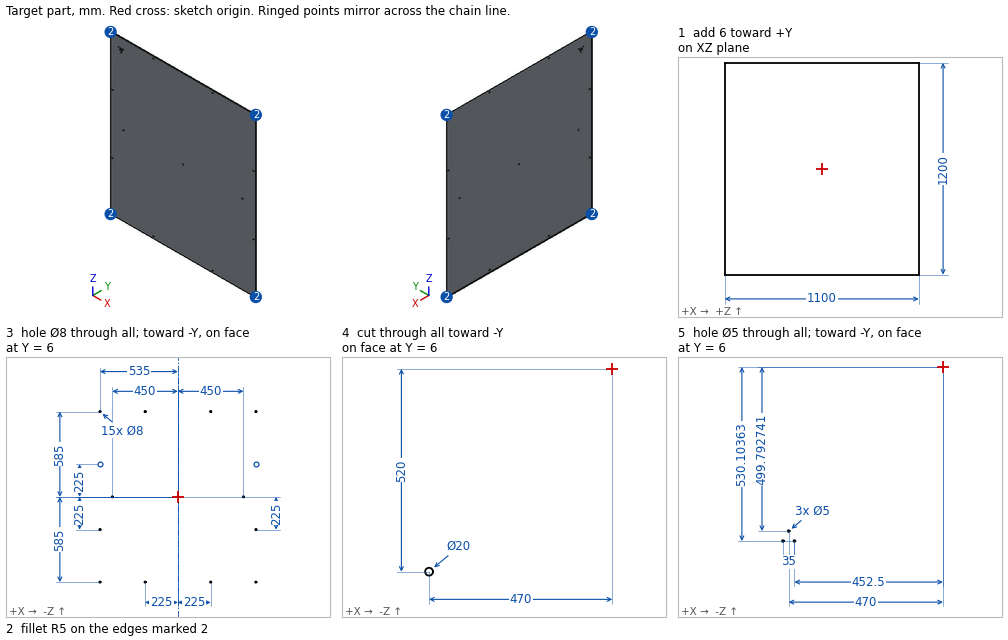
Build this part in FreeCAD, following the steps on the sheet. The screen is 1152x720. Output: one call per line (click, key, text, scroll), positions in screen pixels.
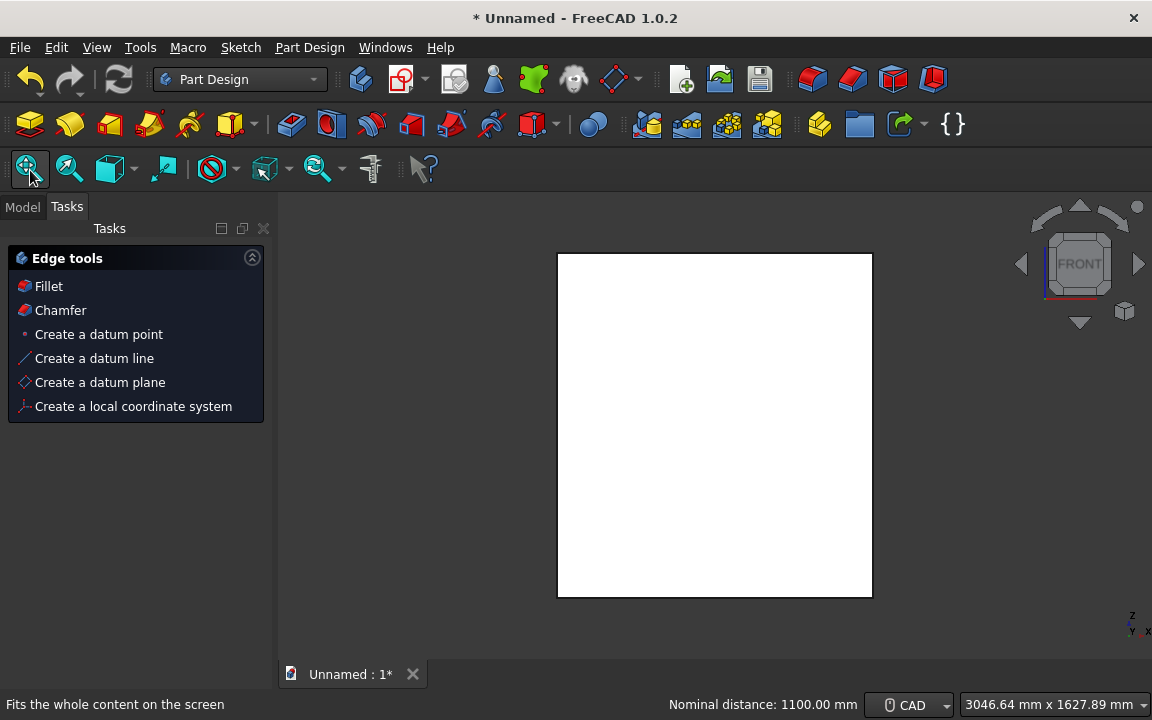
scroll(557, 597, up, 15)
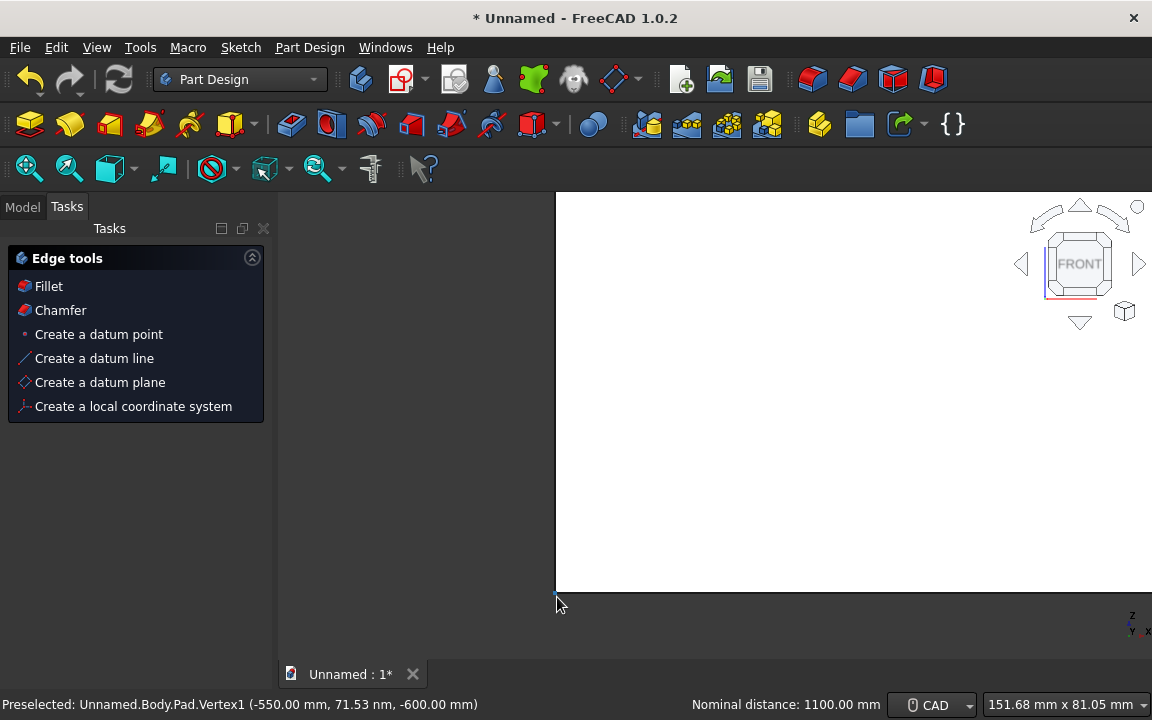
click(30, 170)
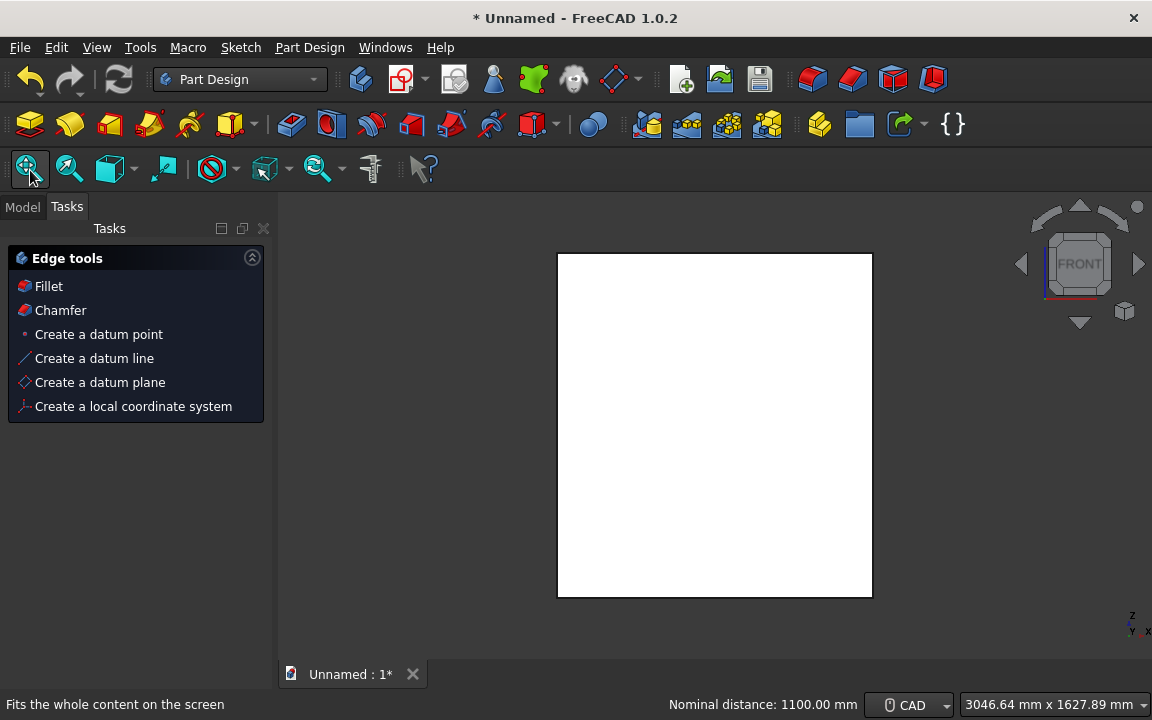
key(3)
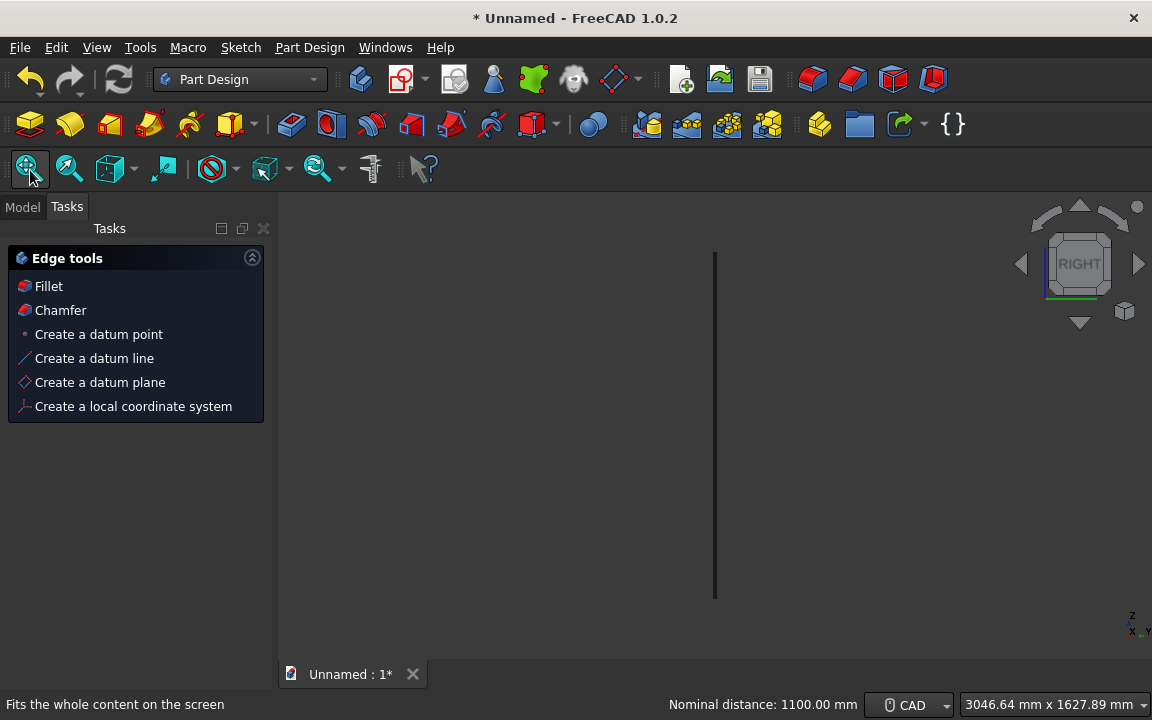
scroll(715, 597, up, 15)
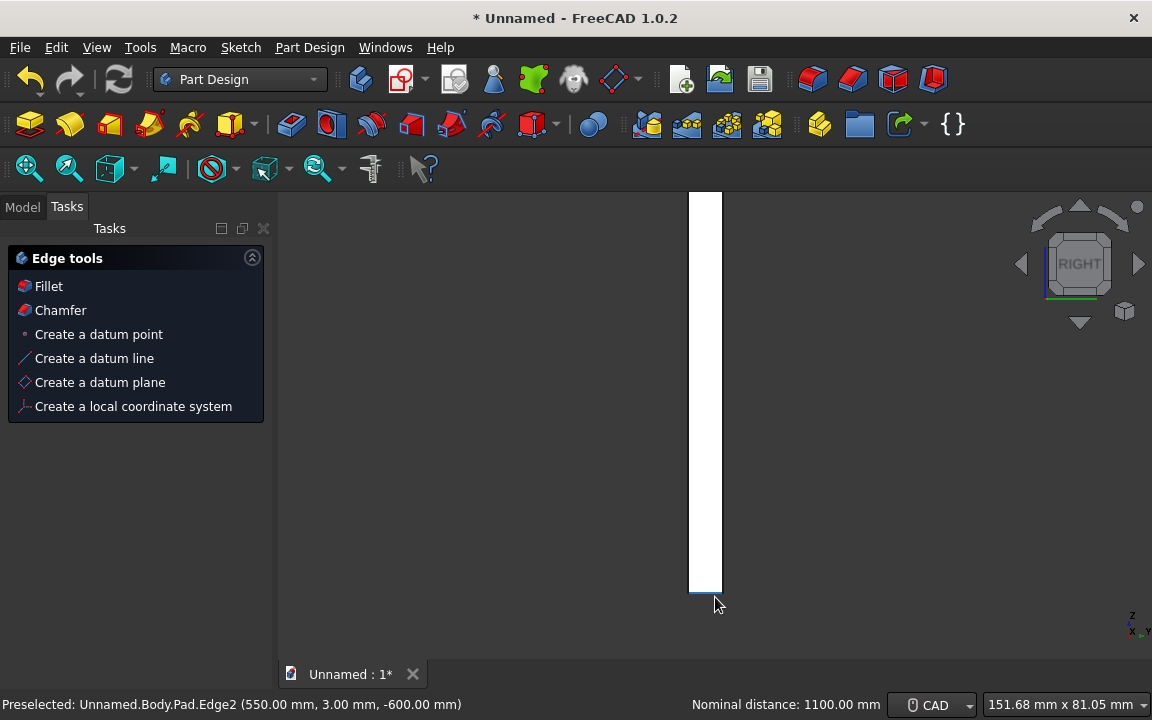
click(705, 592, ctrl)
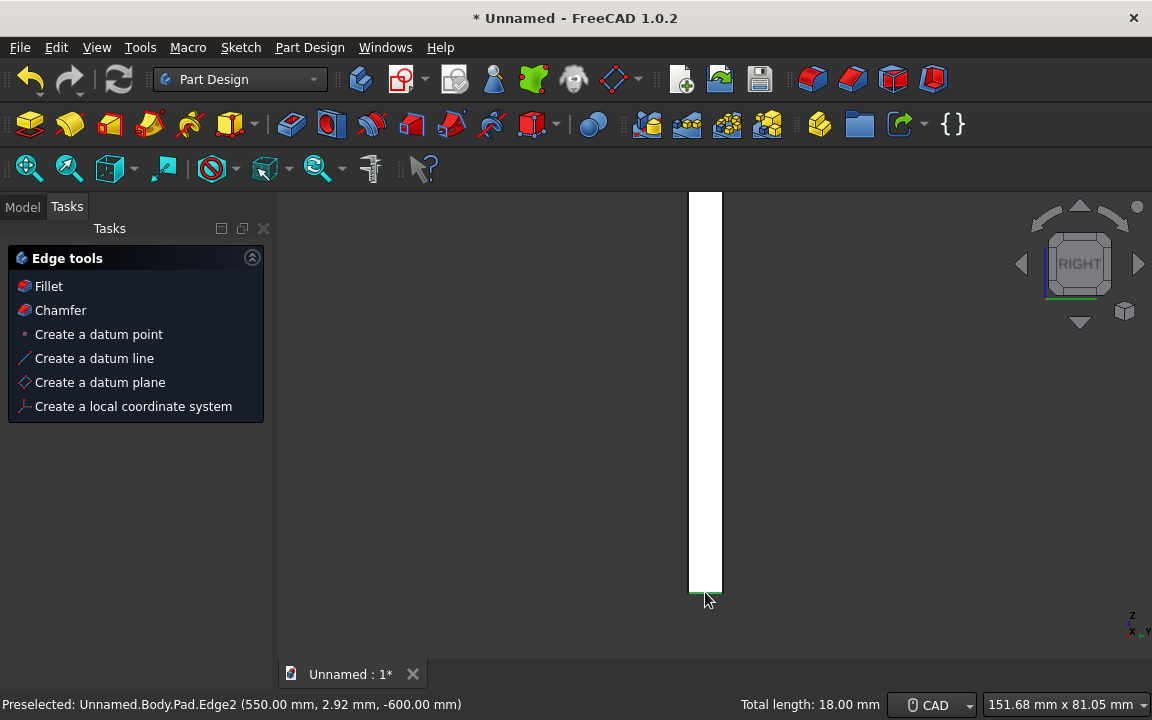
click(30, 170)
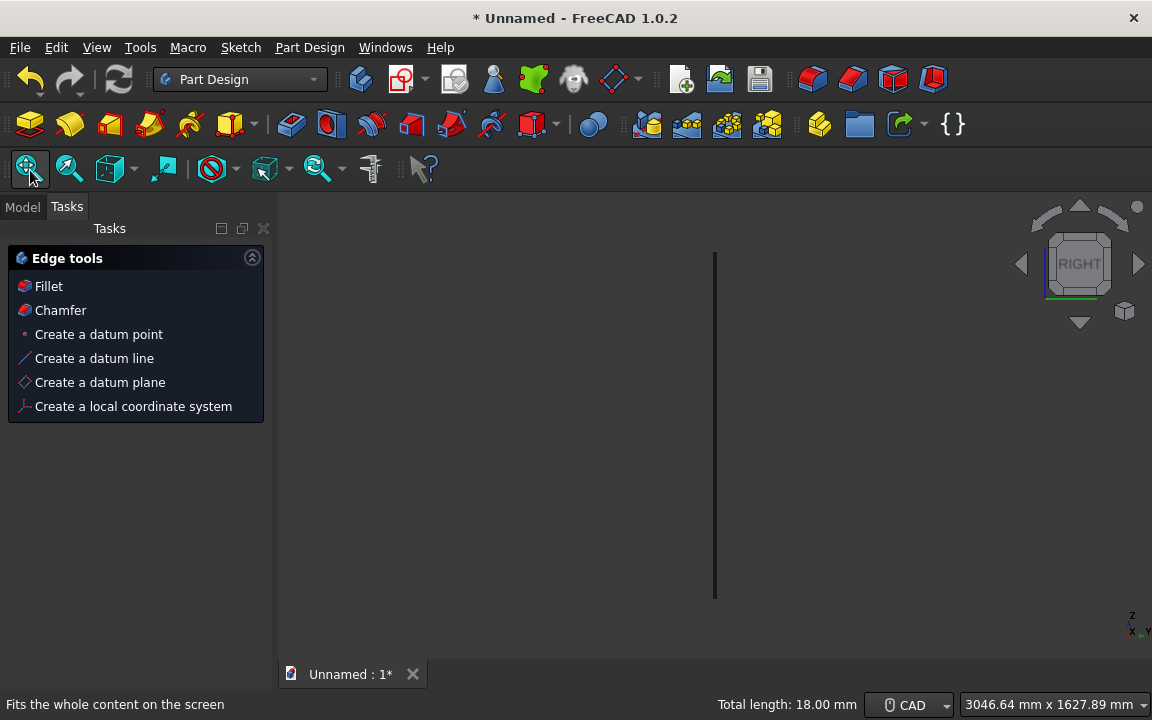
key(5)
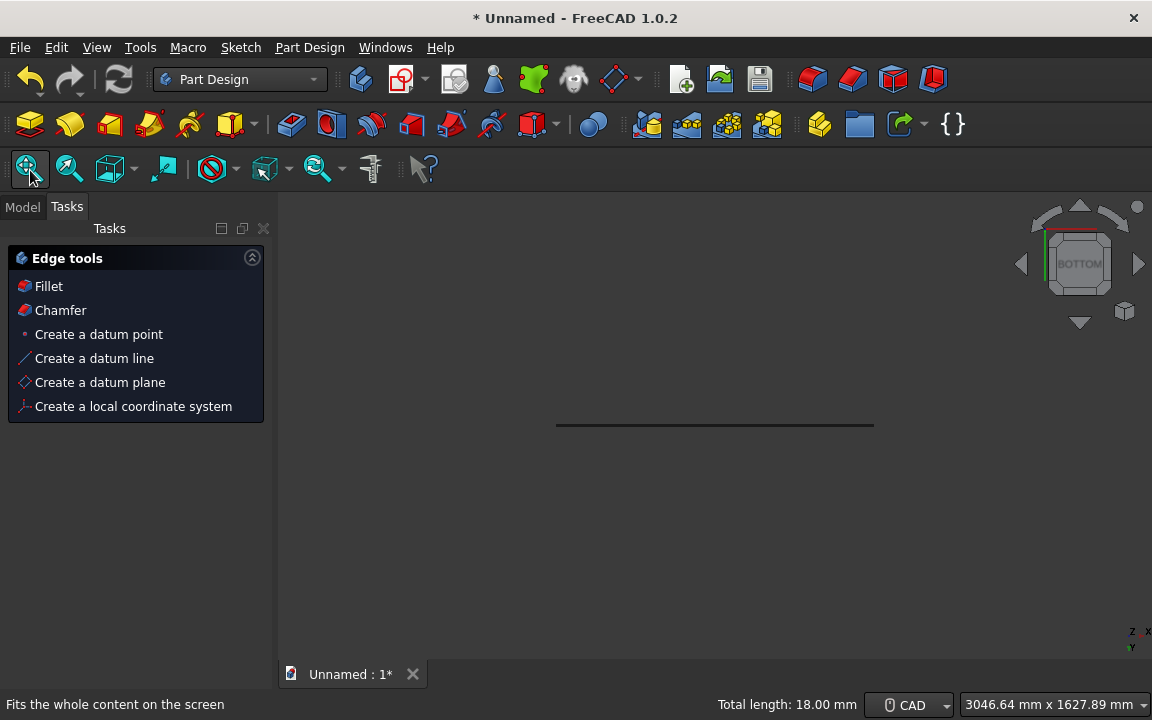
click(30, 170)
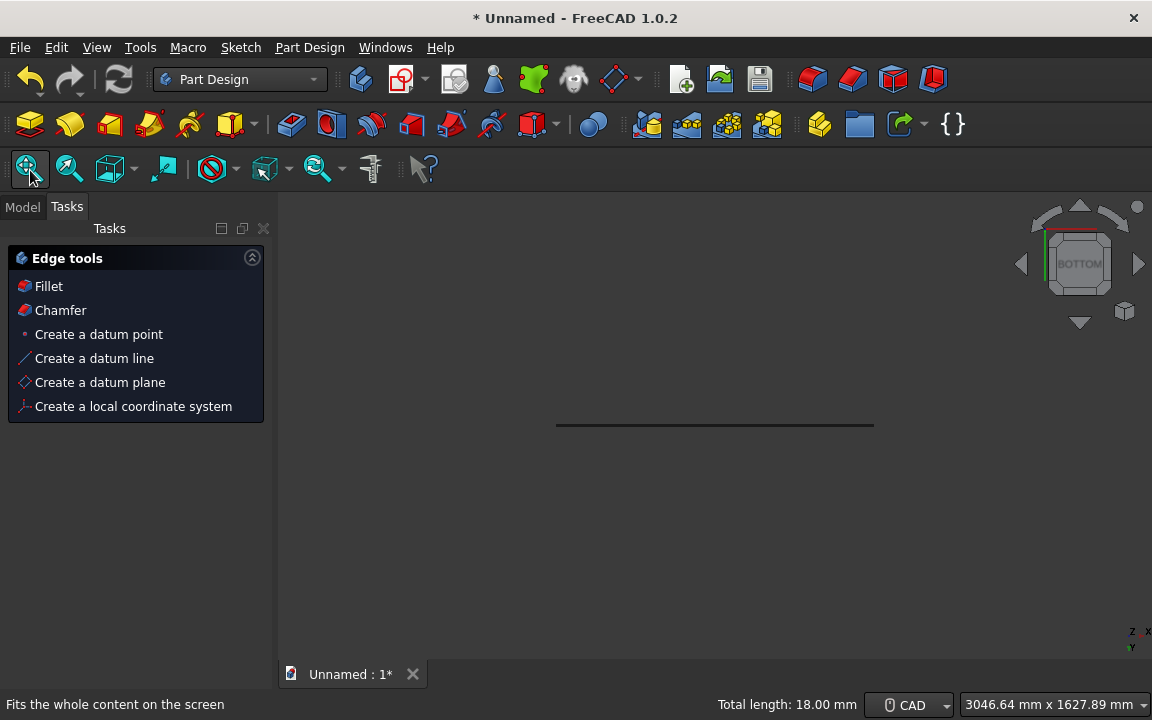
scroll(557, 424, up, 15)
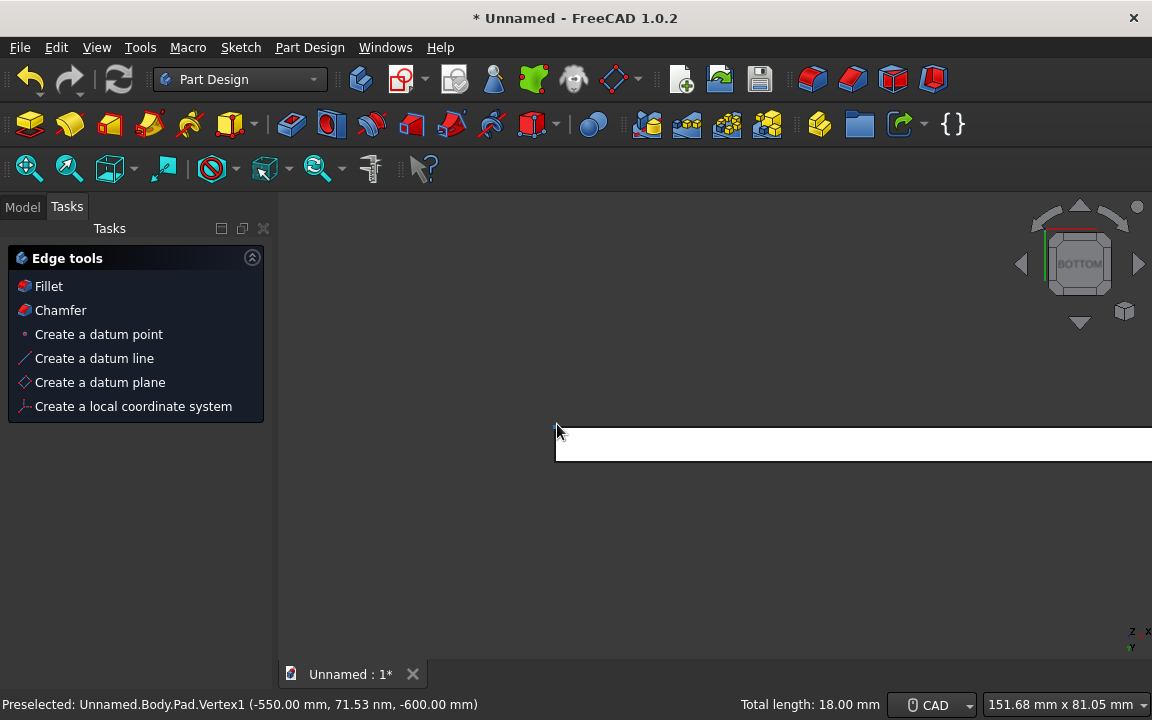
click(555, 444, ctrl)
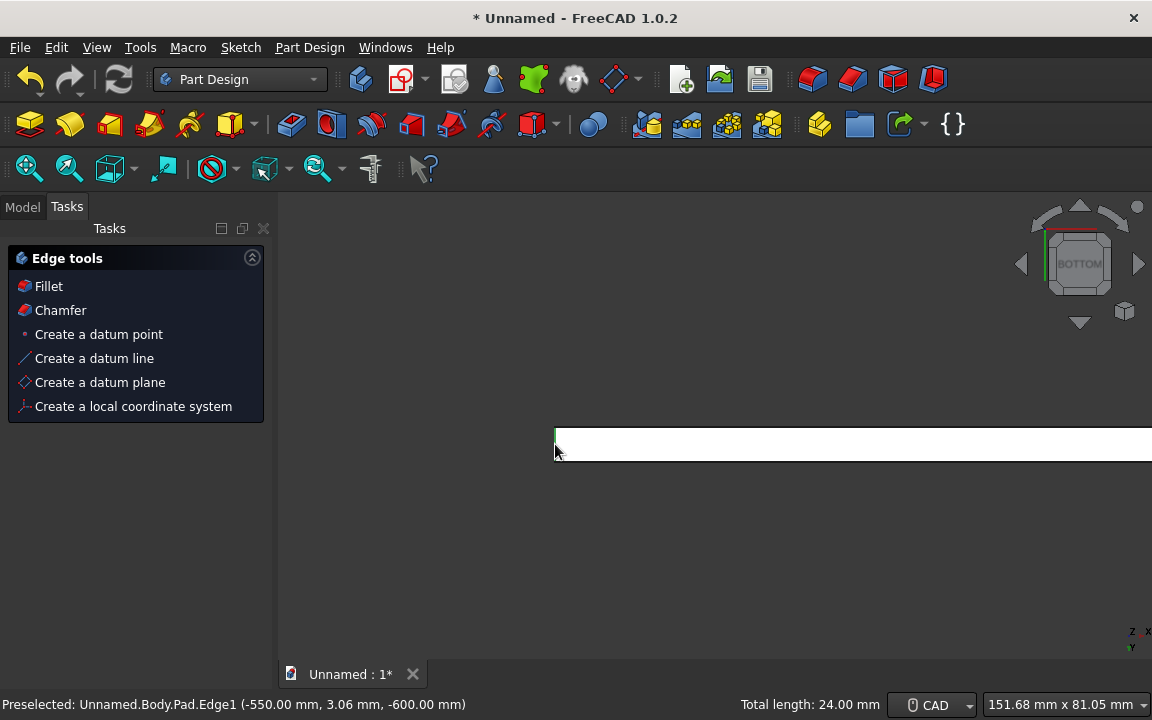
click(814, 80)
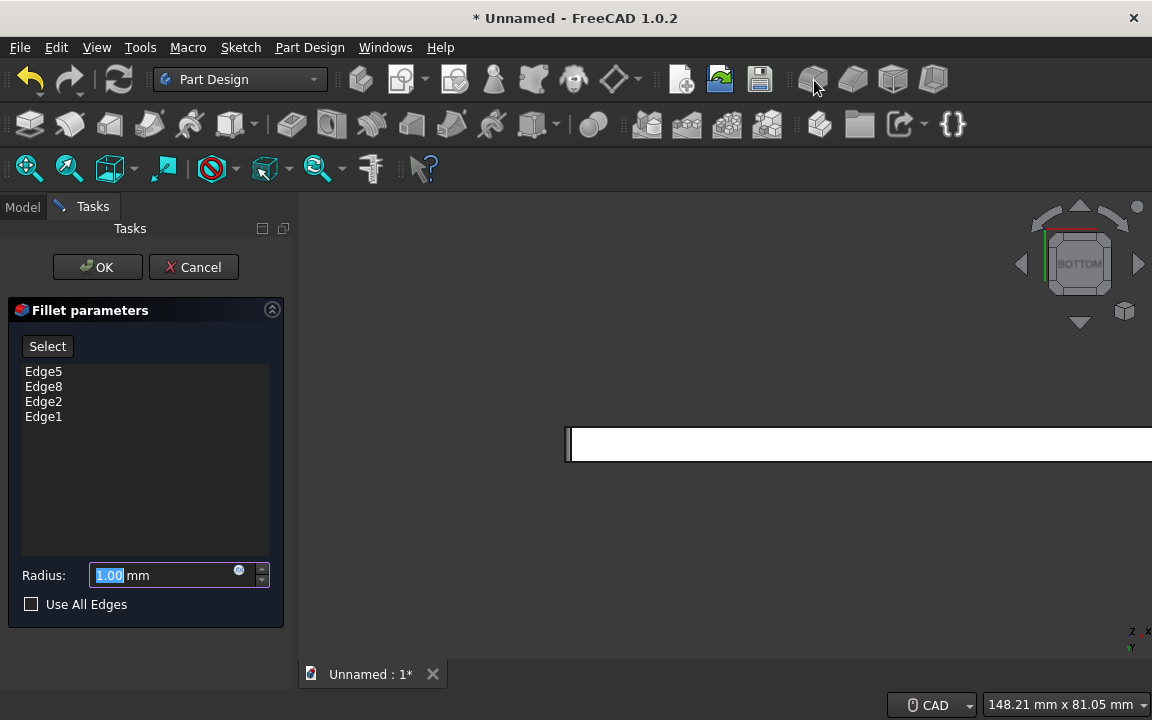
text(5)
key(Tab)